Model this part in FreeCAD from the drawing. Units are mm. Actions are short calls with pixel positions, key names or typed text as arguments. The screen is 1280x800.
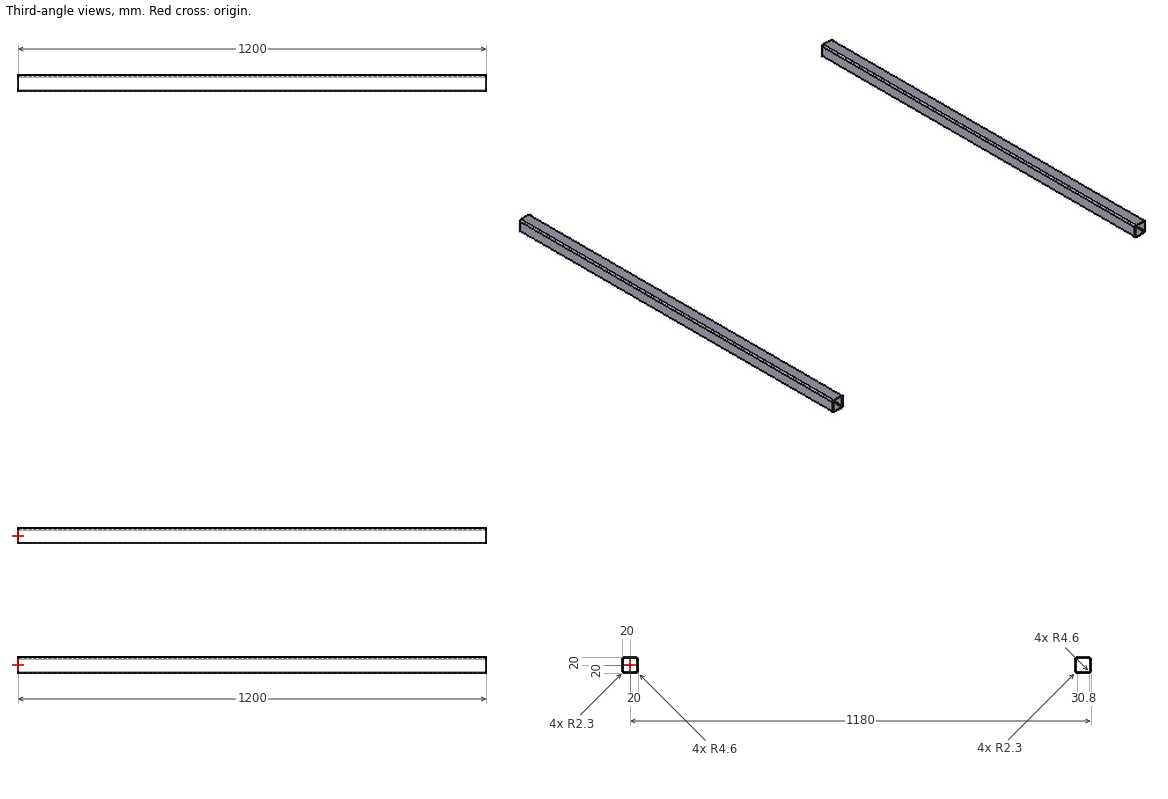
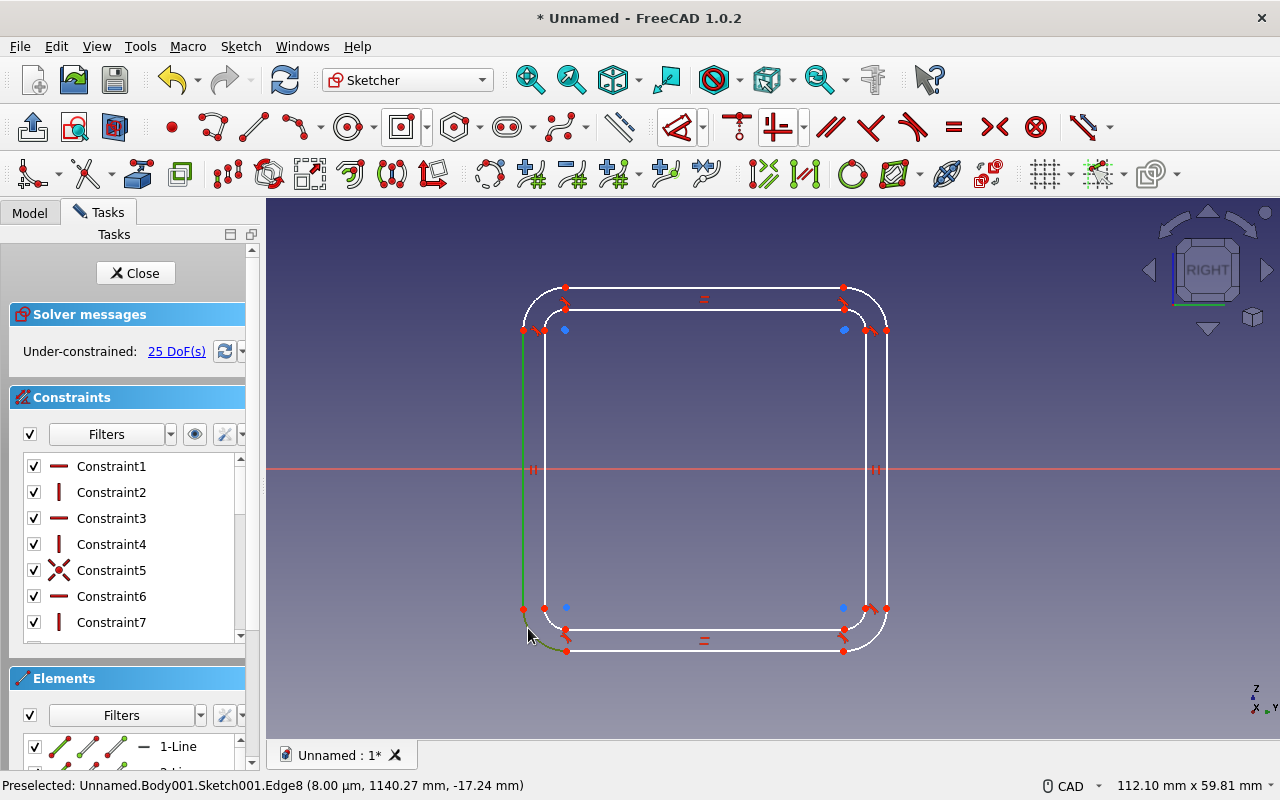
key(t)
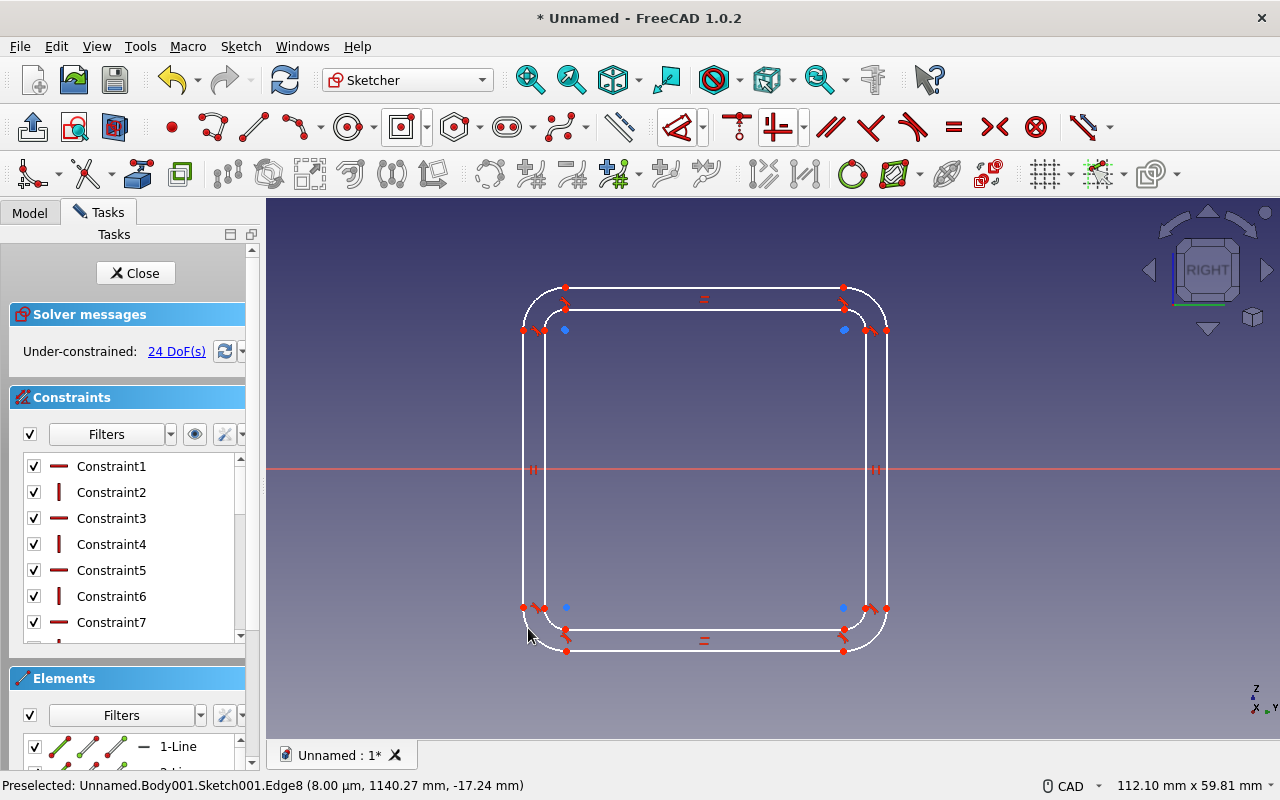
click(761, 630)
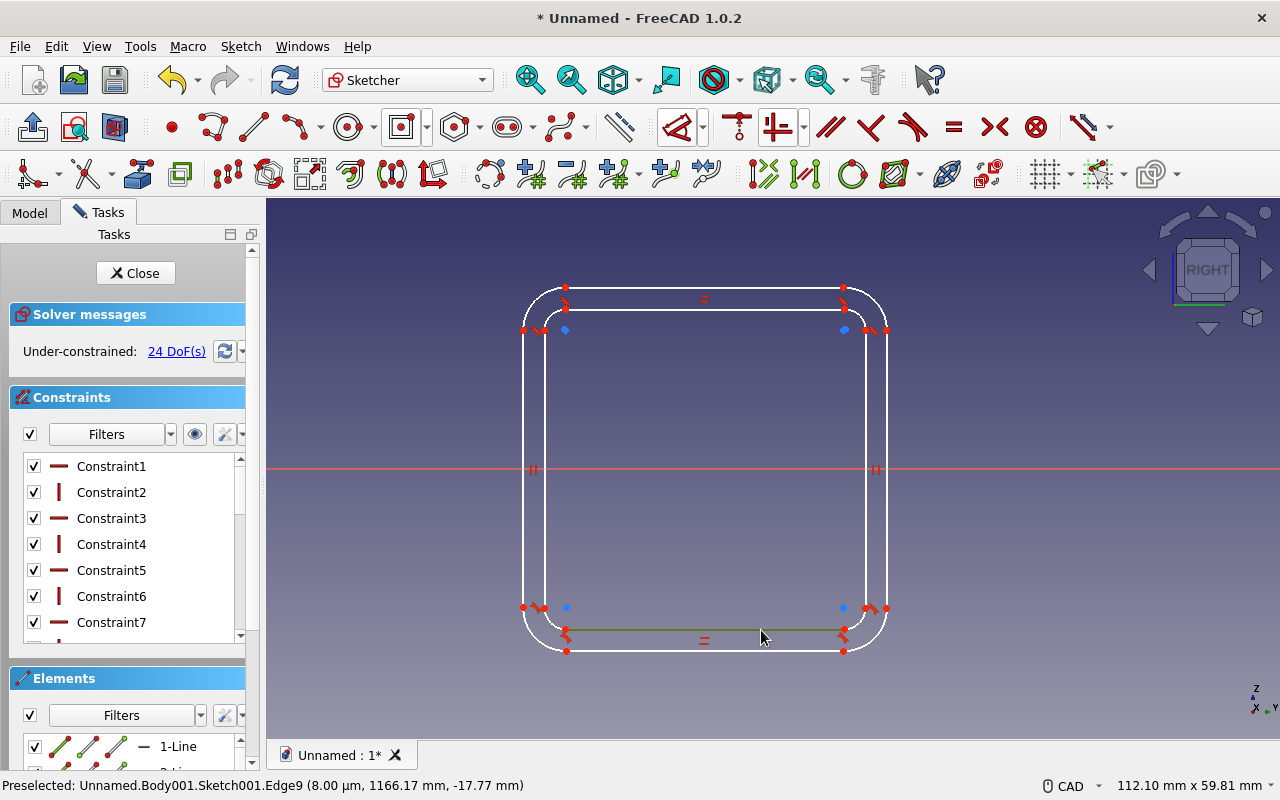
scroll(547, 618, up, 2)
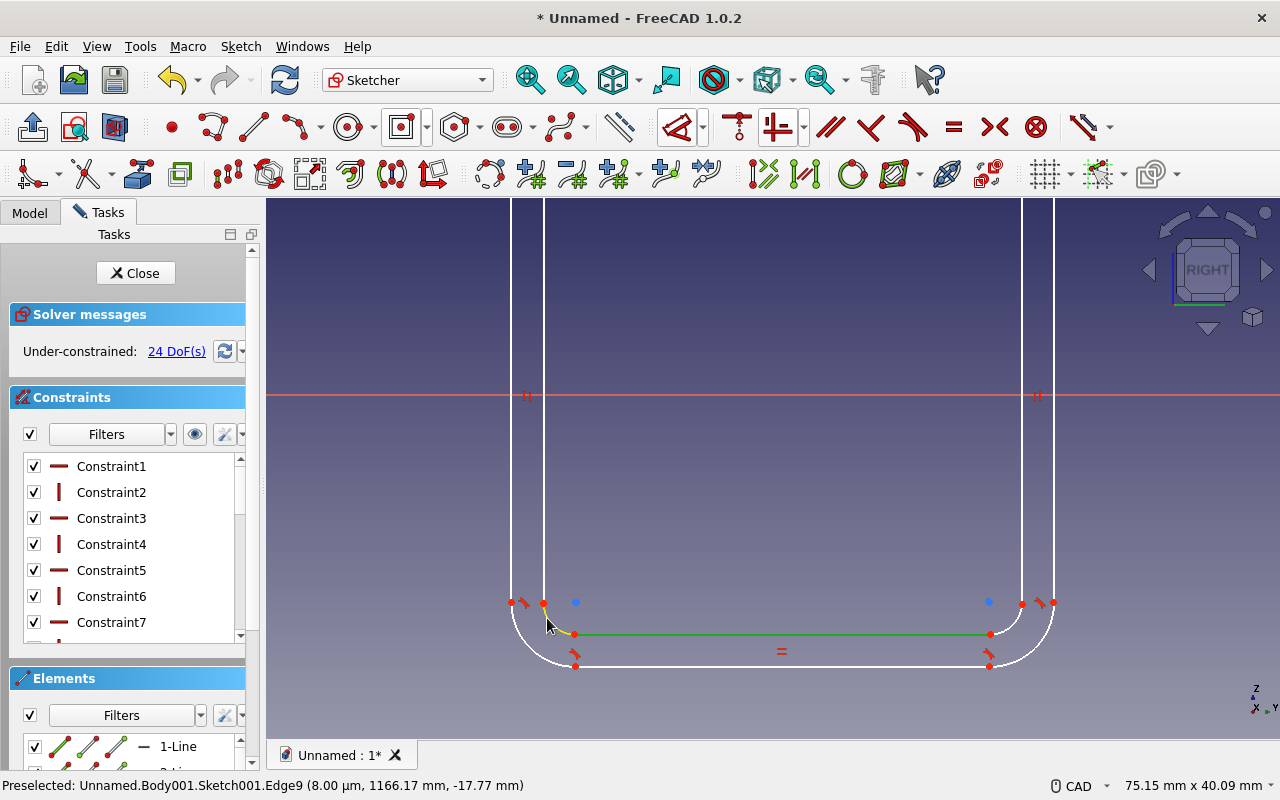
click(547, 618)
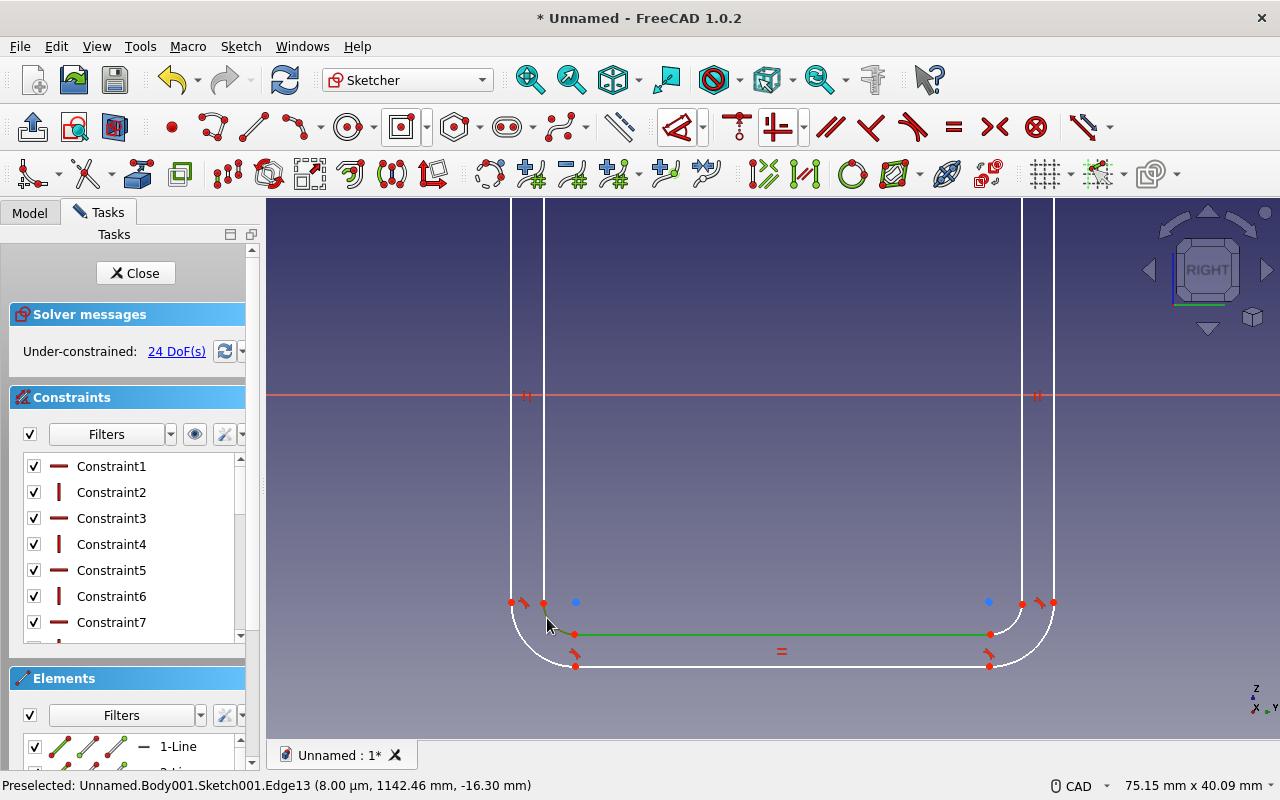
key(t)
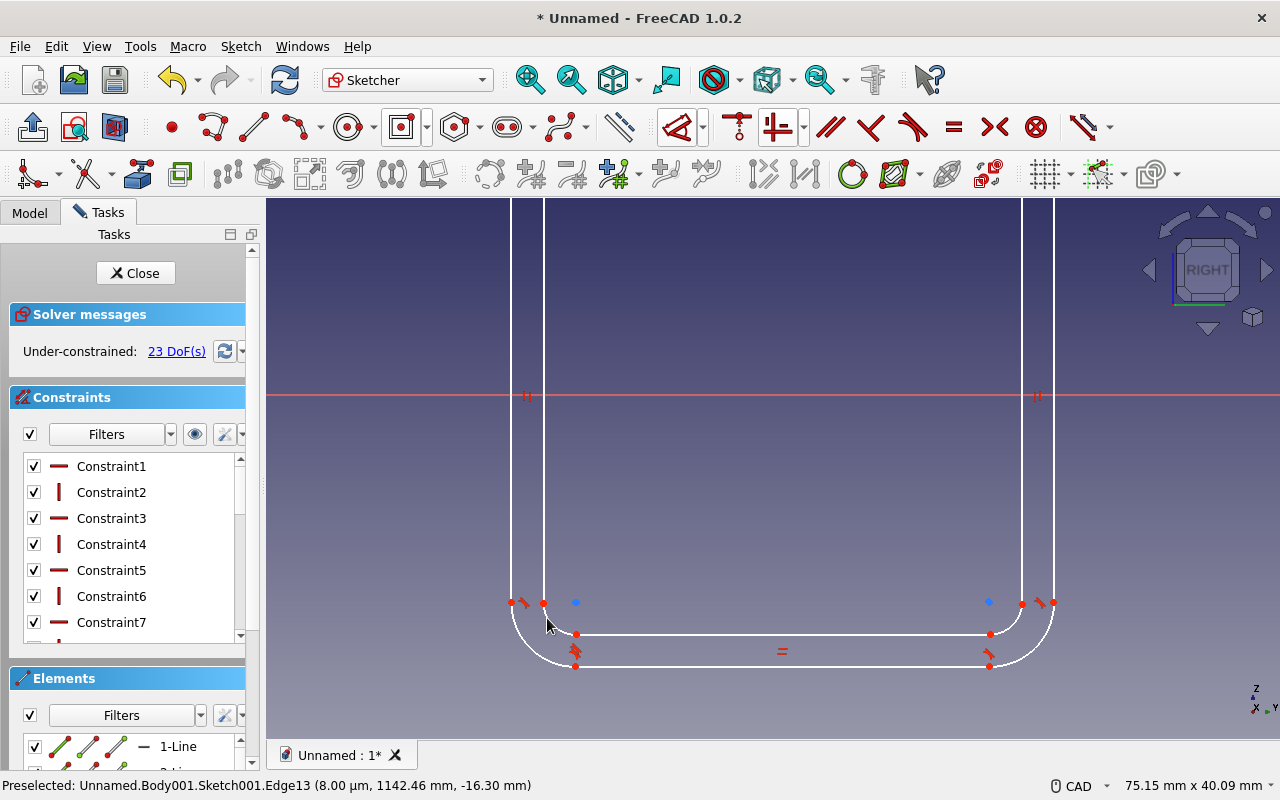
click(866, 635)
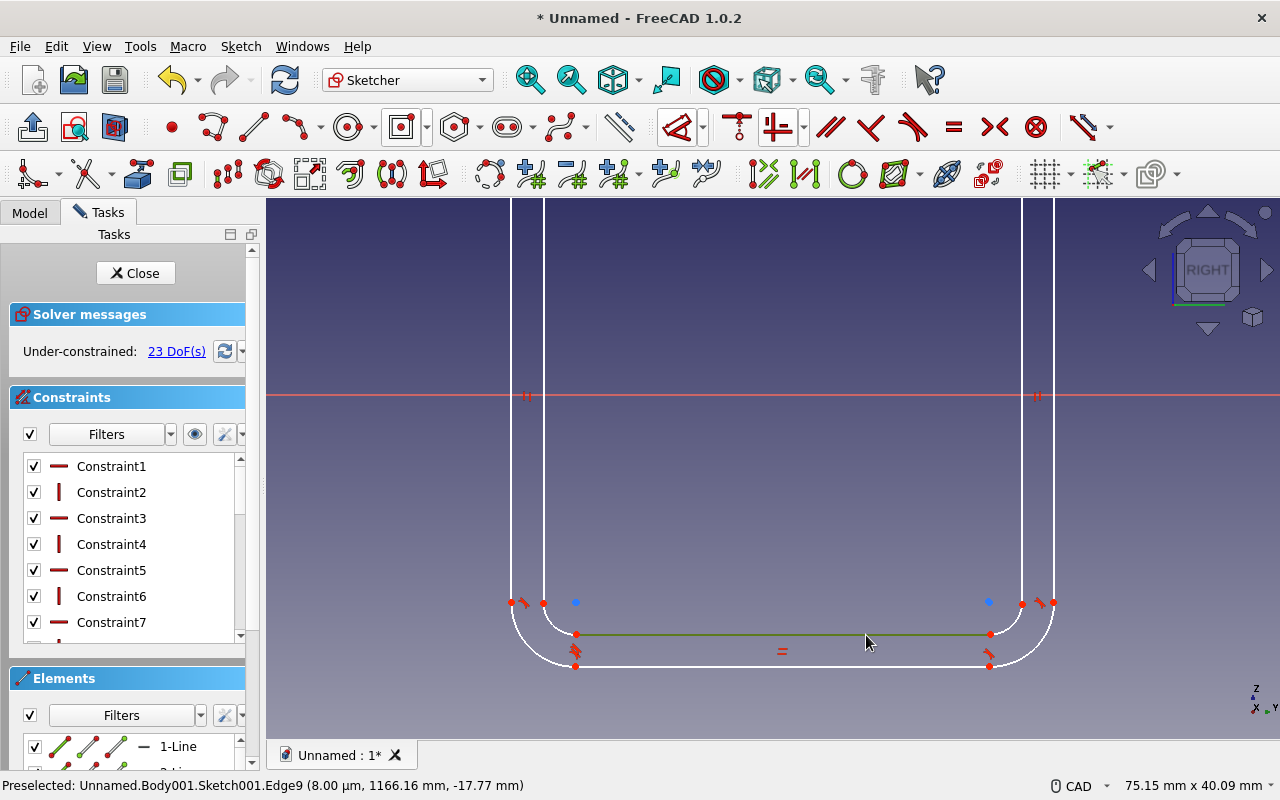
click(1004, 631)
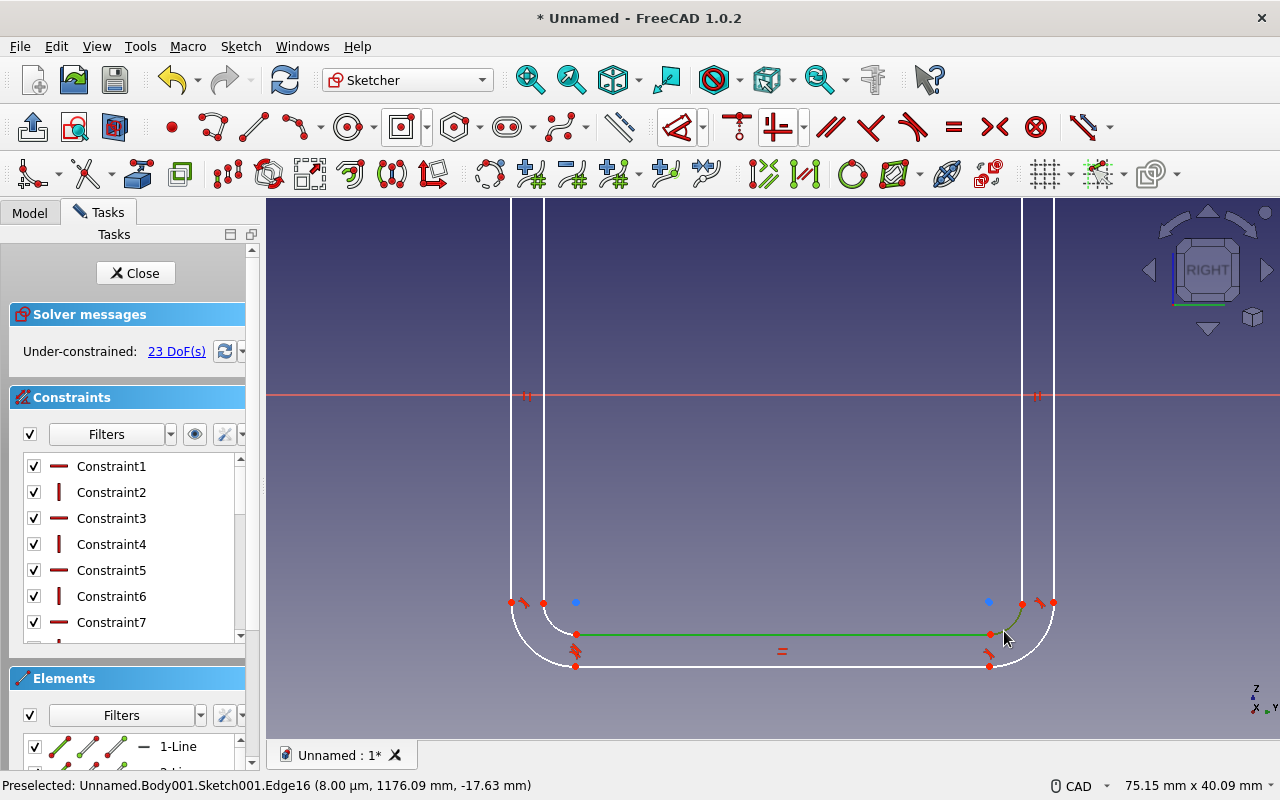
key(t)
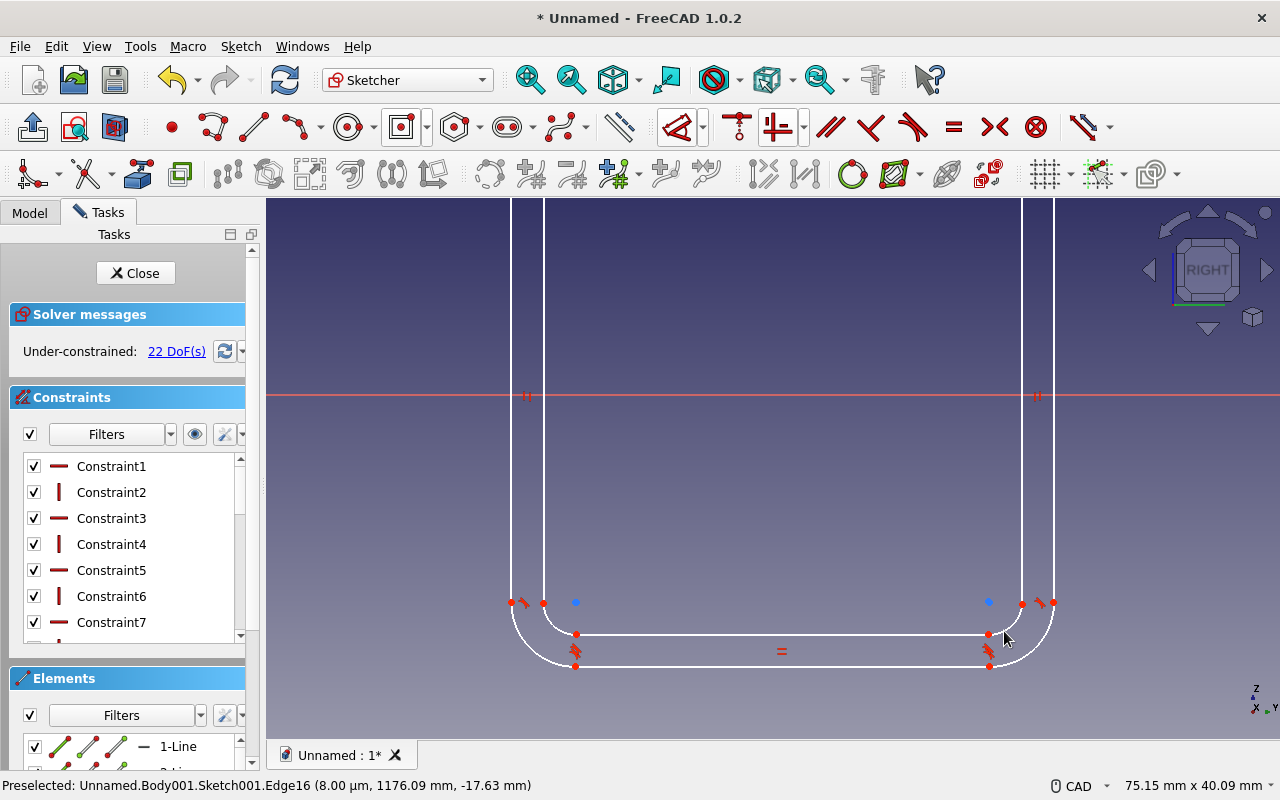
click(544, 480)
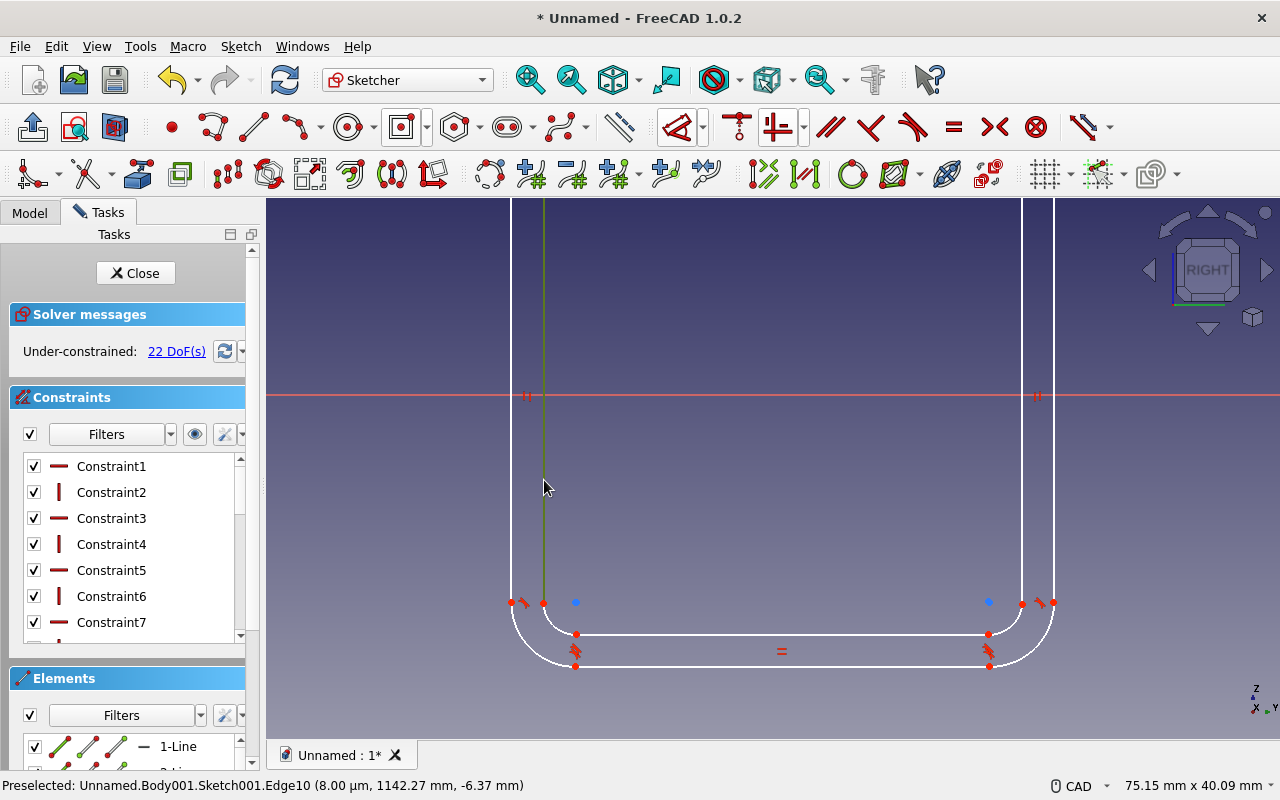
click(548, 618)